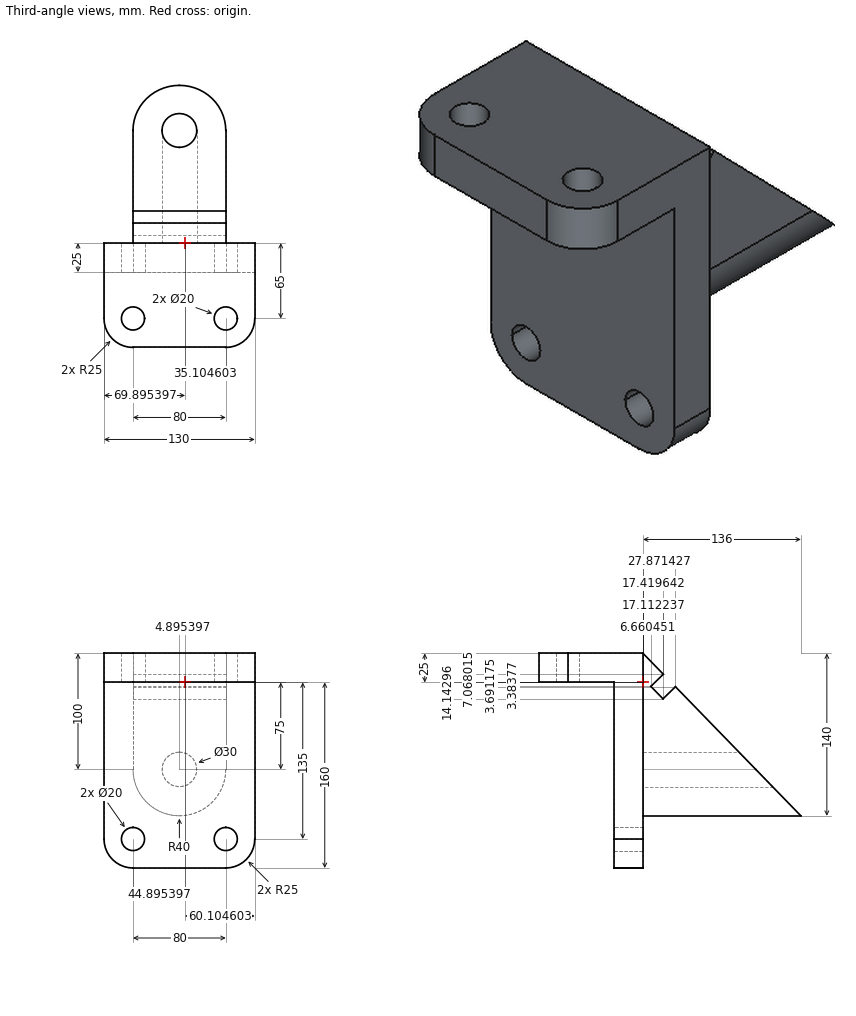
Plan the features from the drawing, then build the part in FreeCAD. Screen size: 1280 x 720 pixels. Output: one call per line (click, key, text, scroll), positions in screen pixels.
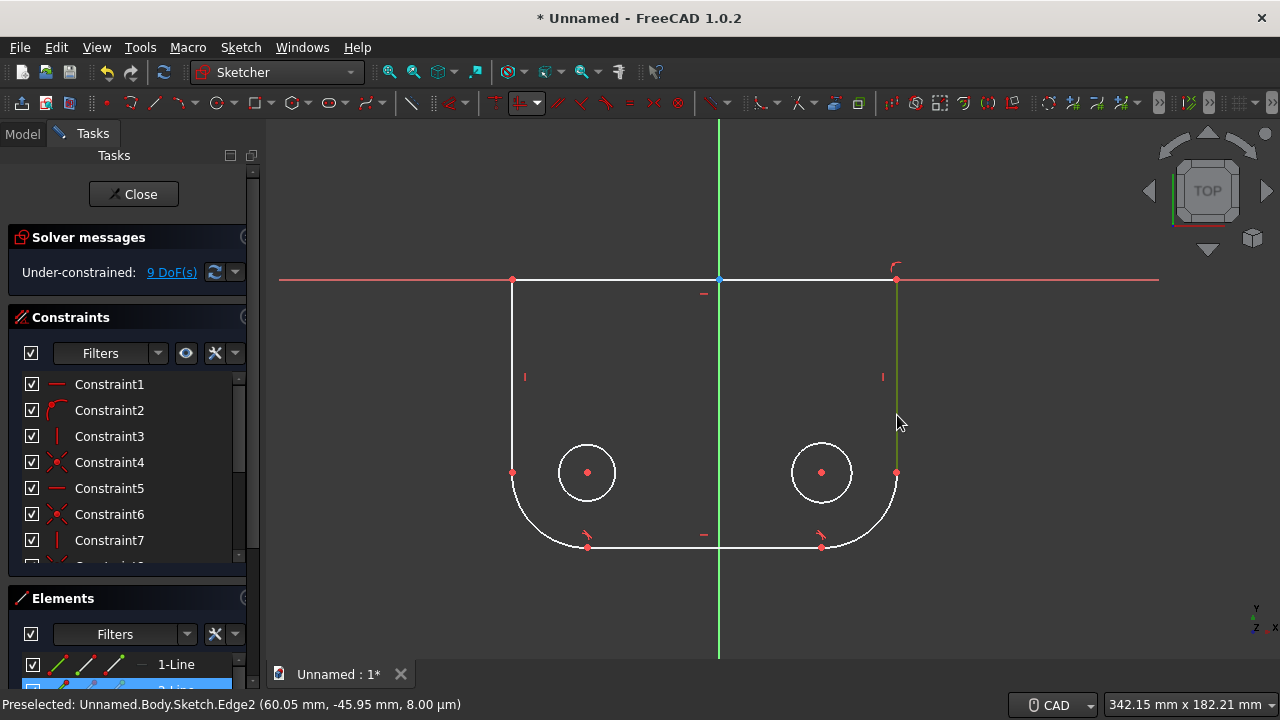
click(856, 540)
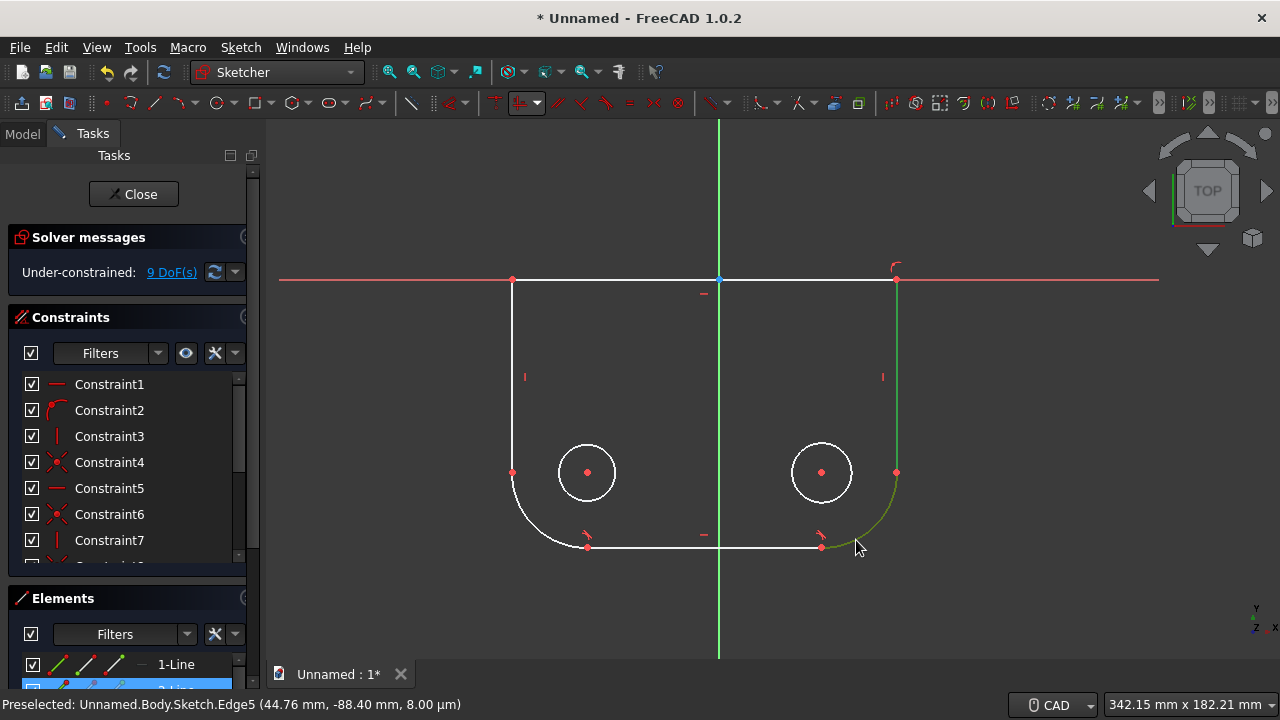
click(606, 104)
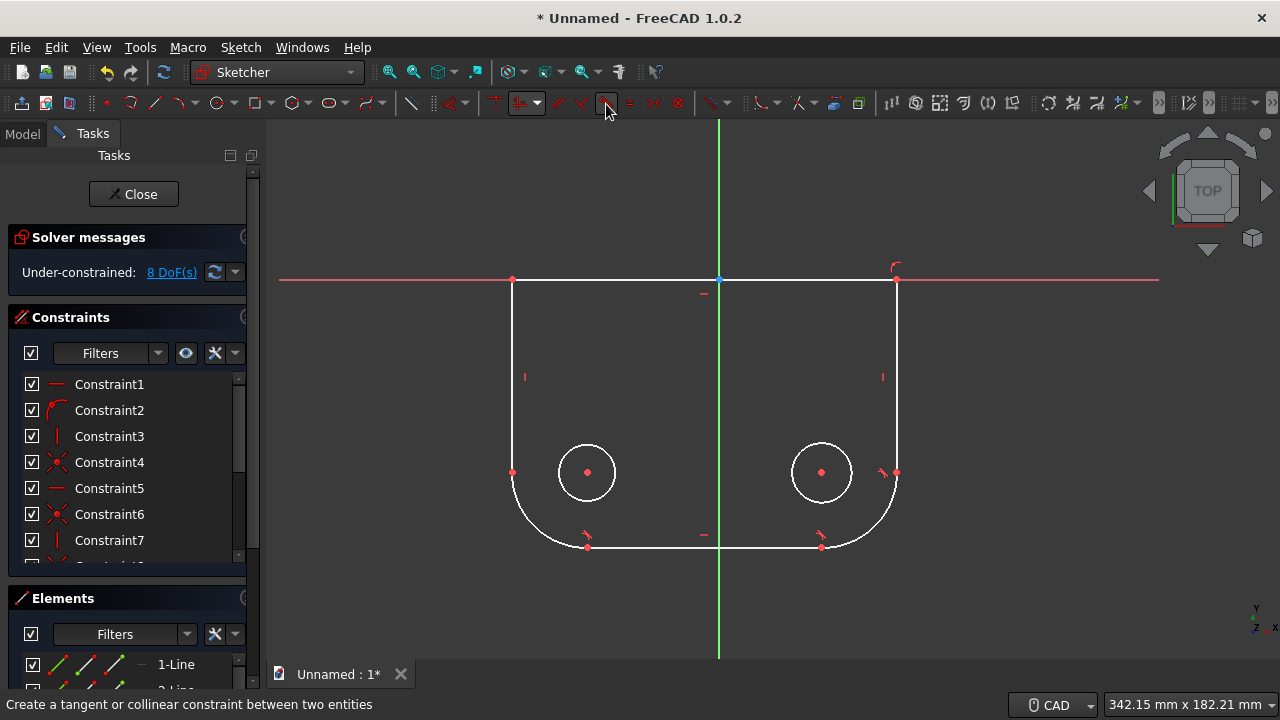
click(512, 338)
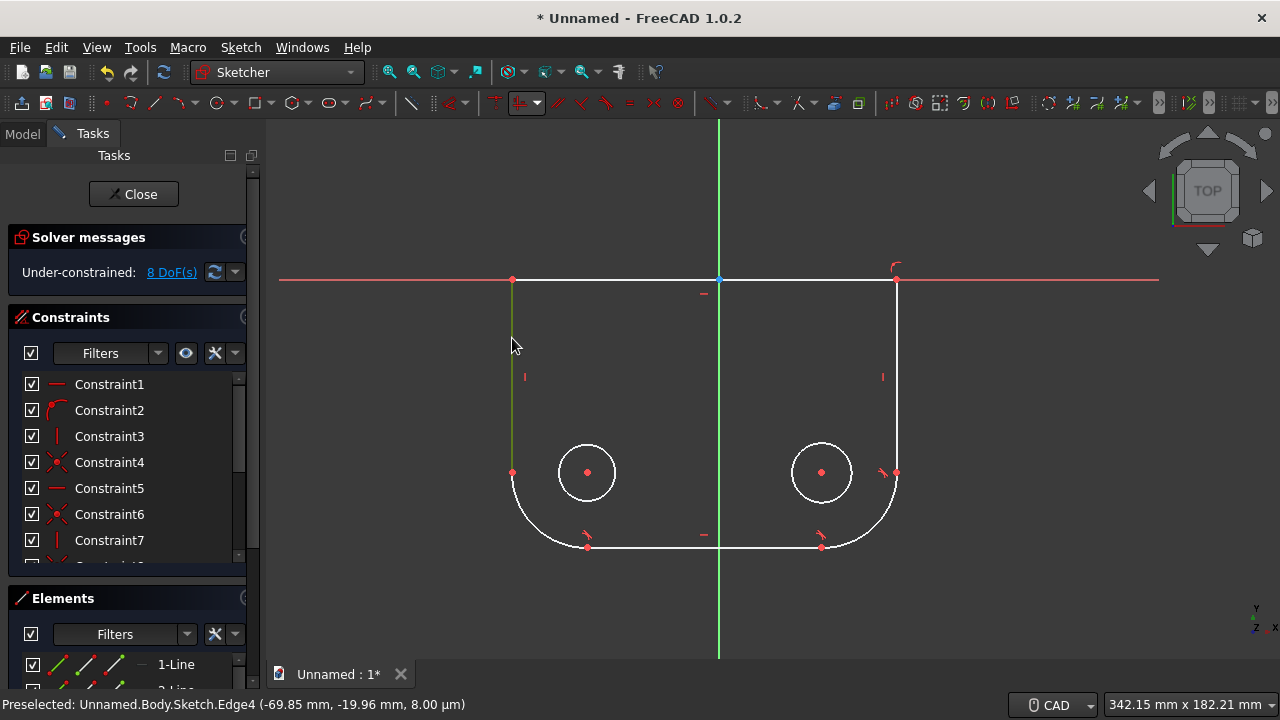
click(520, 507)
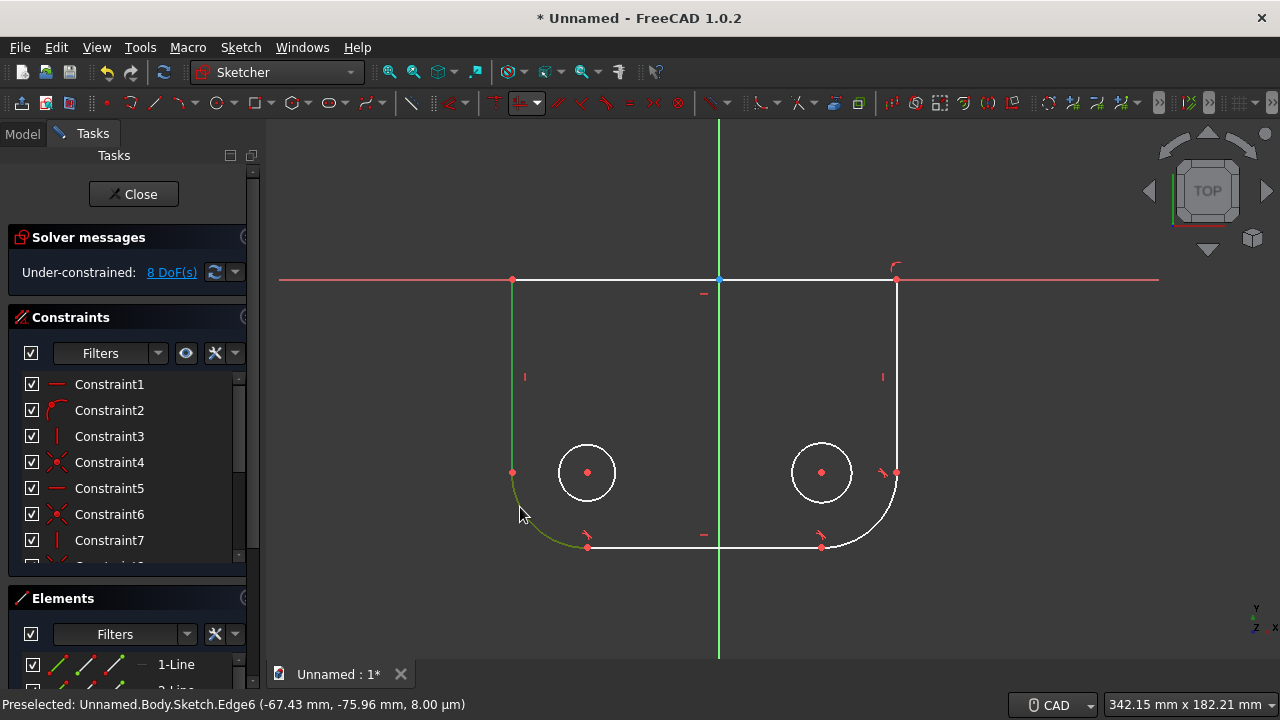
click(606, 104)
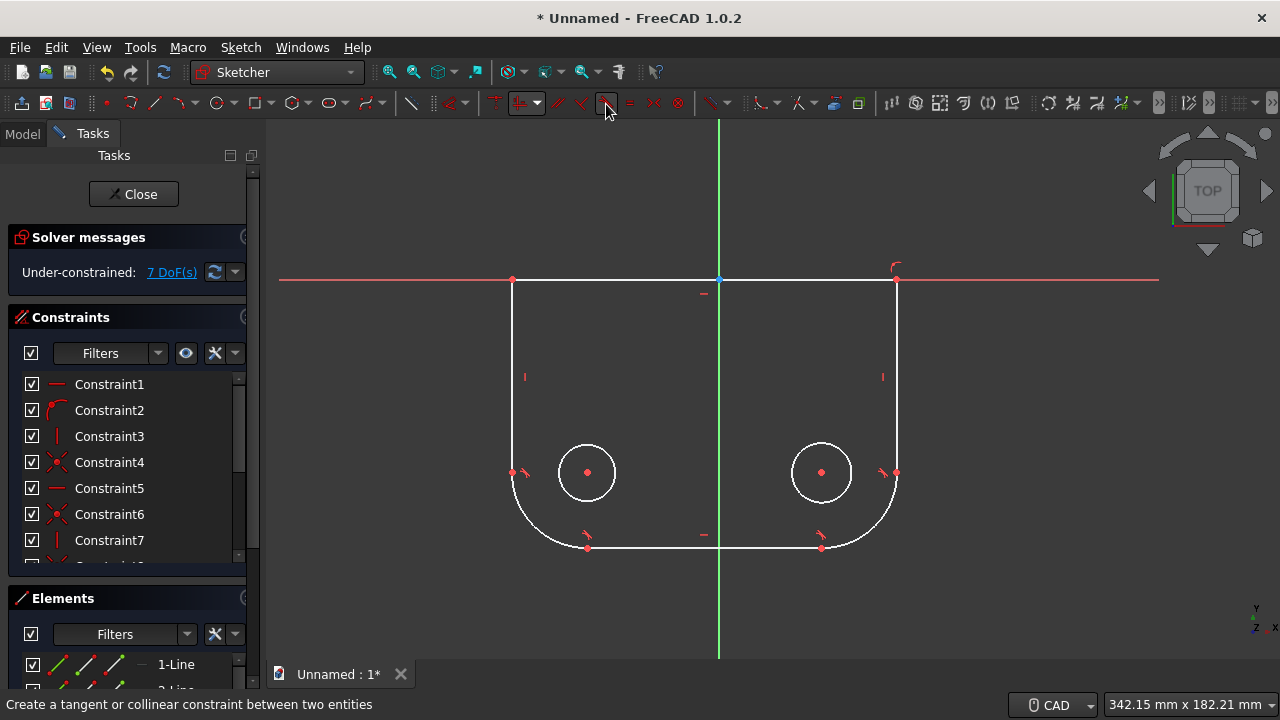
click(856, 540)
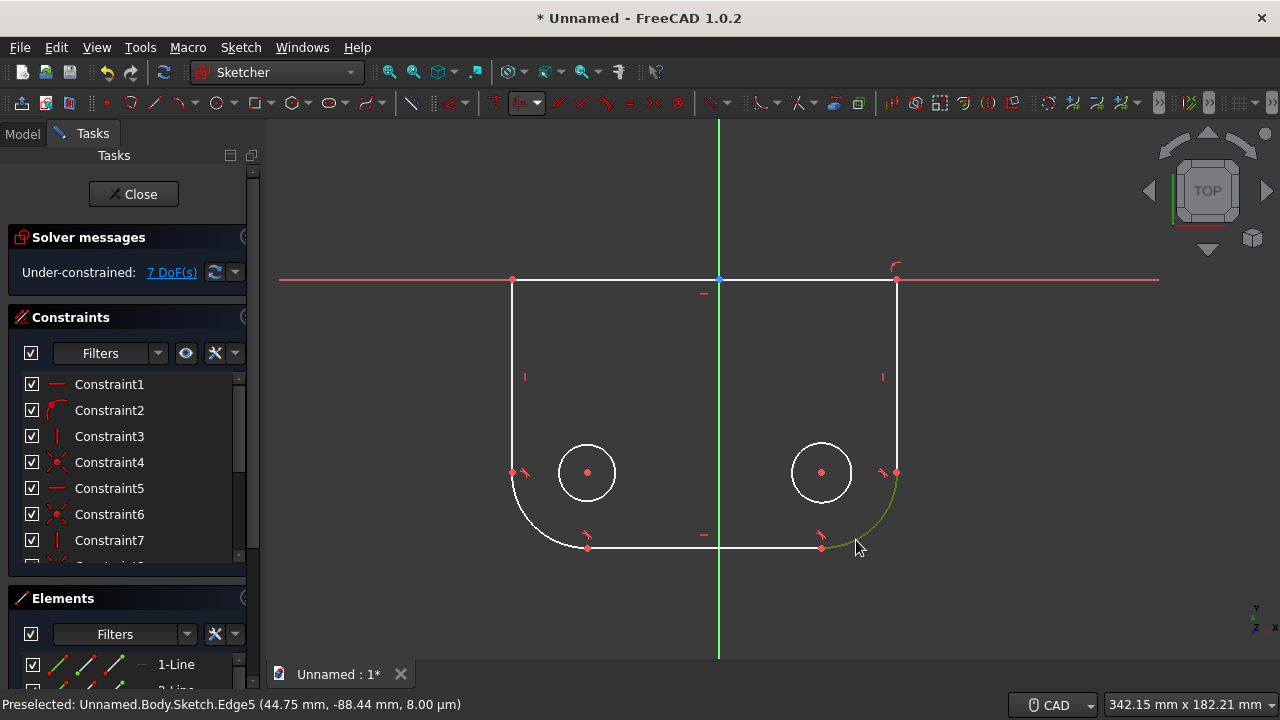
click(520, 507)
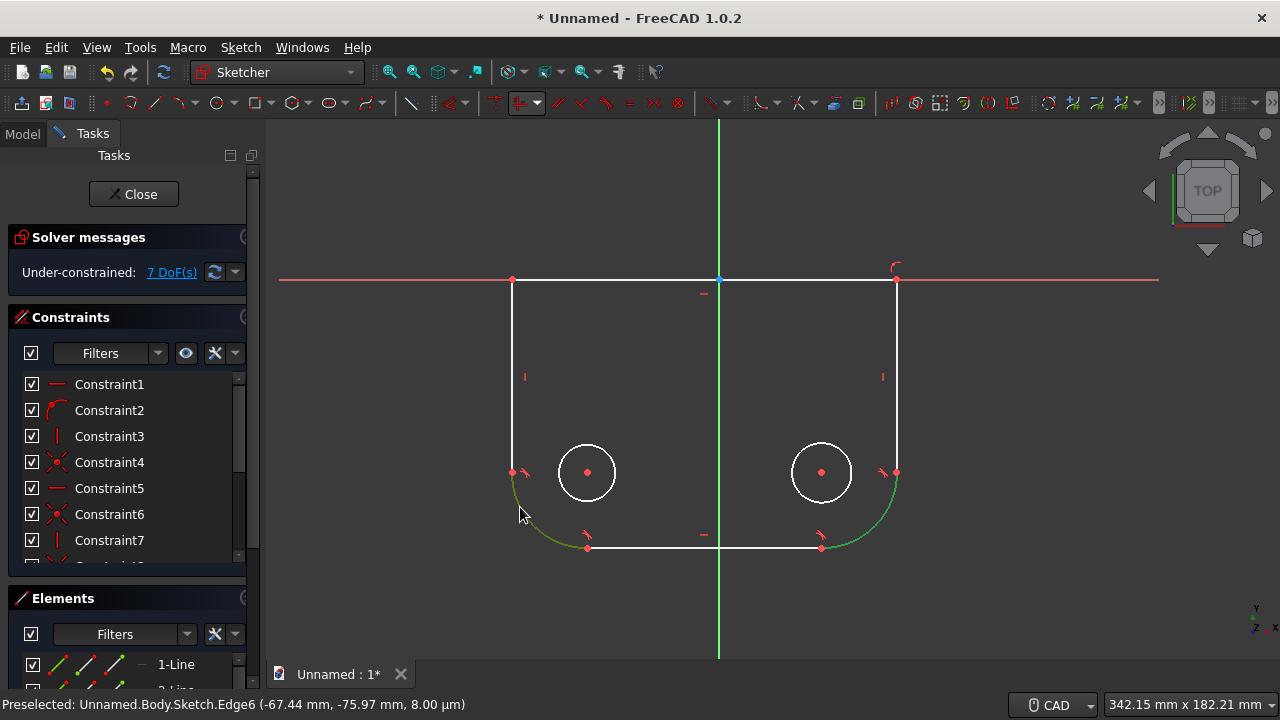
key(e)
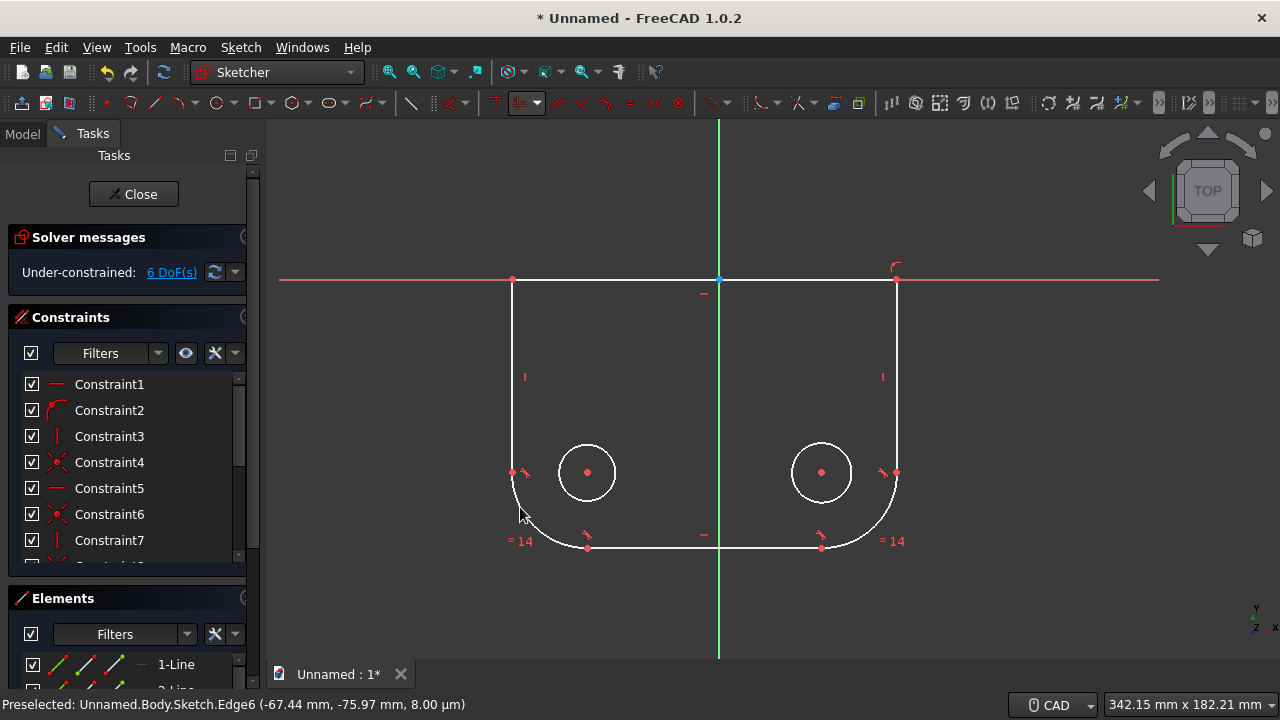
click(843, 452)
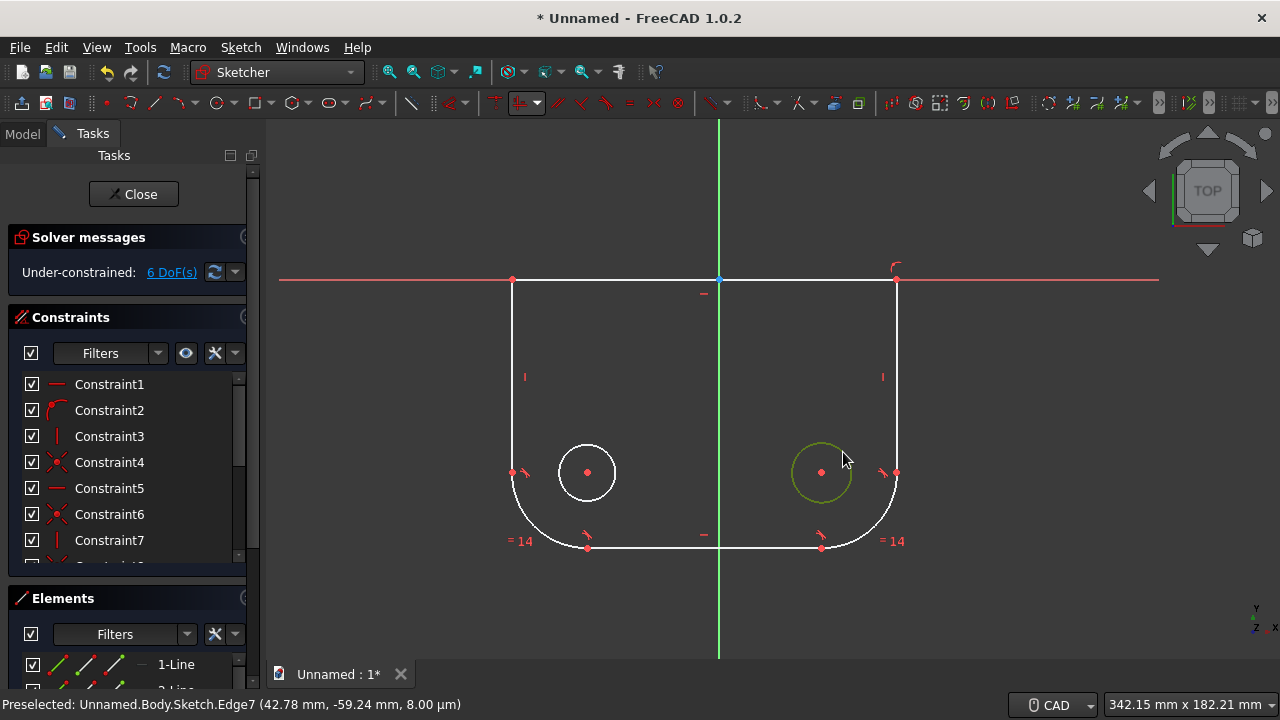
click(607, 453)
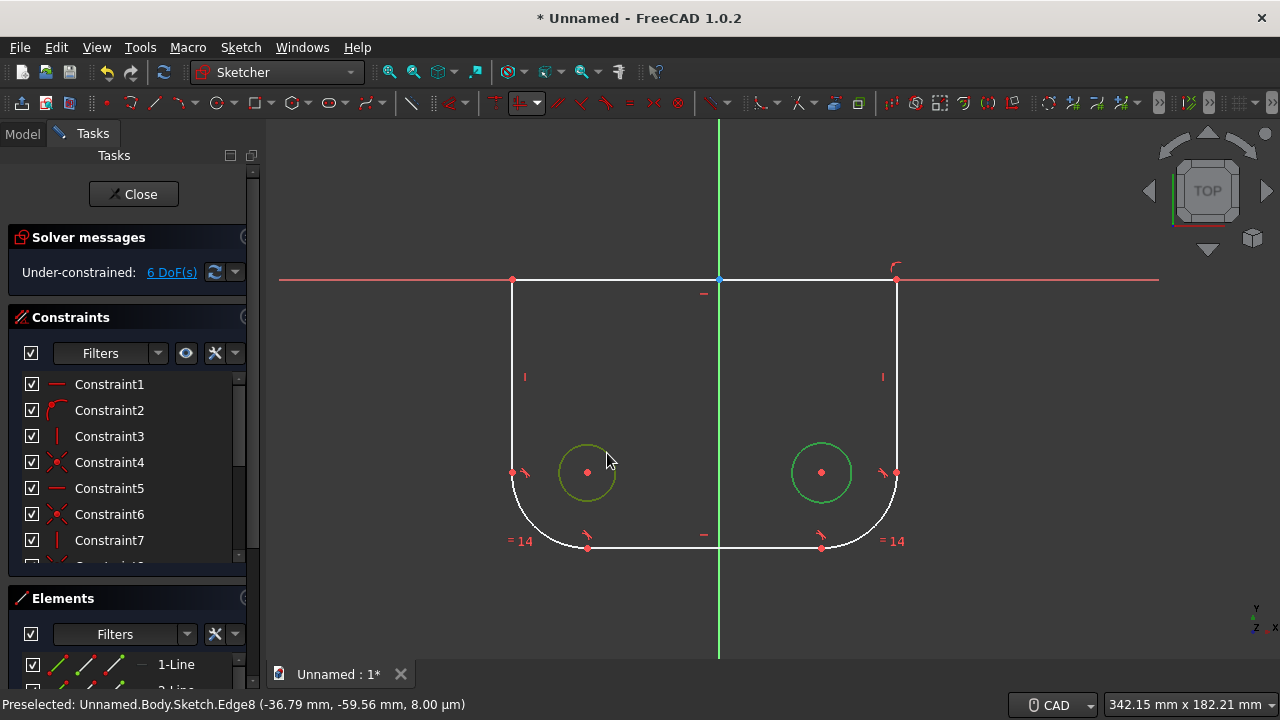
key(e)